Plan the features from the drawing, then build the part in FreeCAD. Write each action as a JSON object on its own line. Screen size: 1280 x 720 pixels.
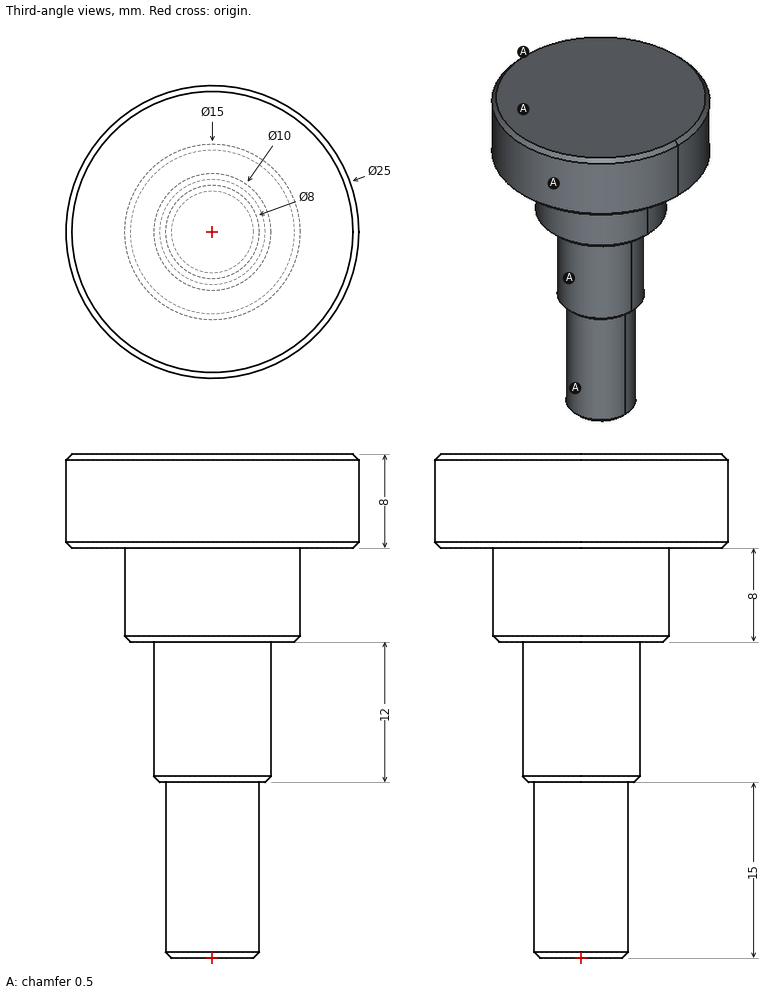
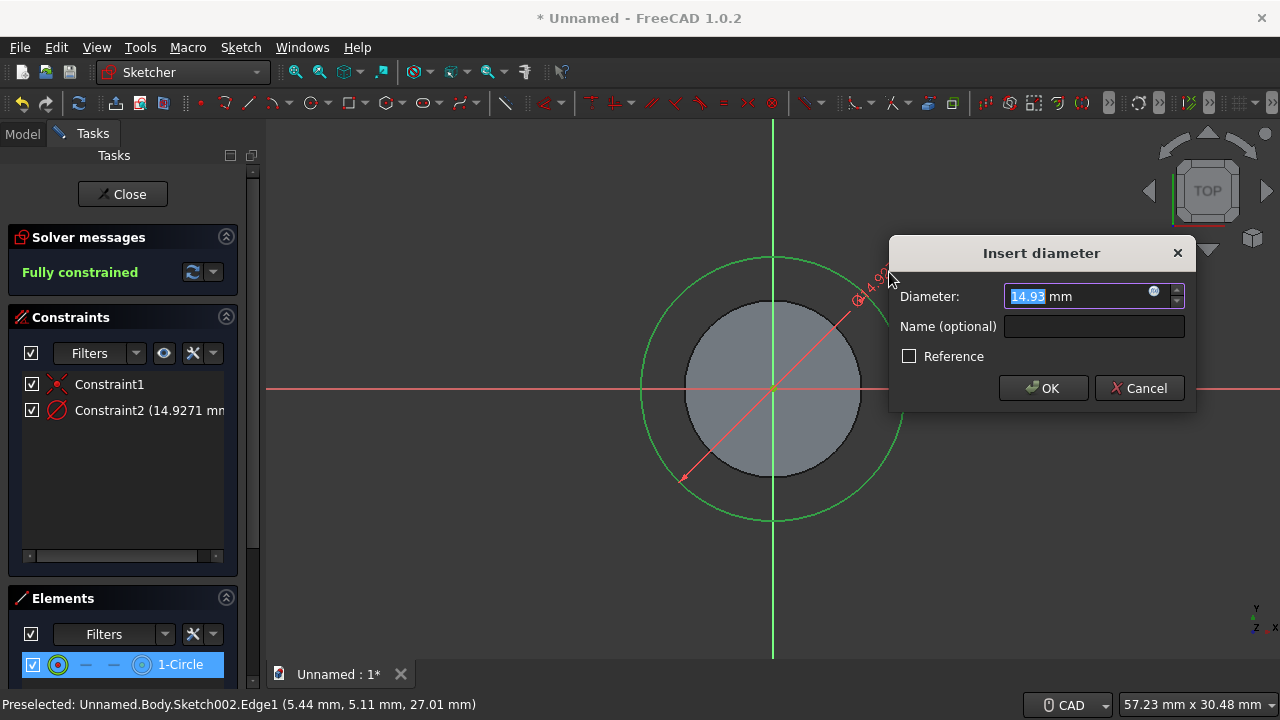
{"action": "type", "text": "15"}
{"action": "key", "text": "Return"}
{"action": "key", "text": "Escape"}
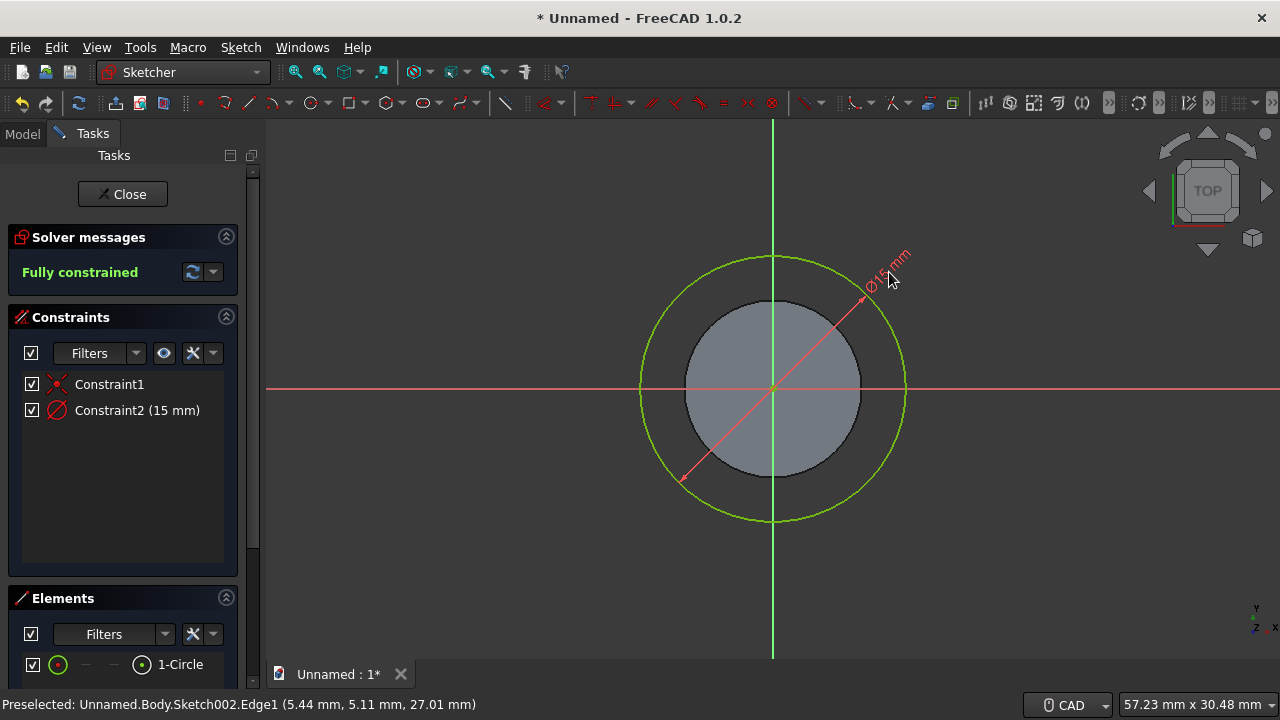
{"action": "left_click", "coordinate": [123, 194]}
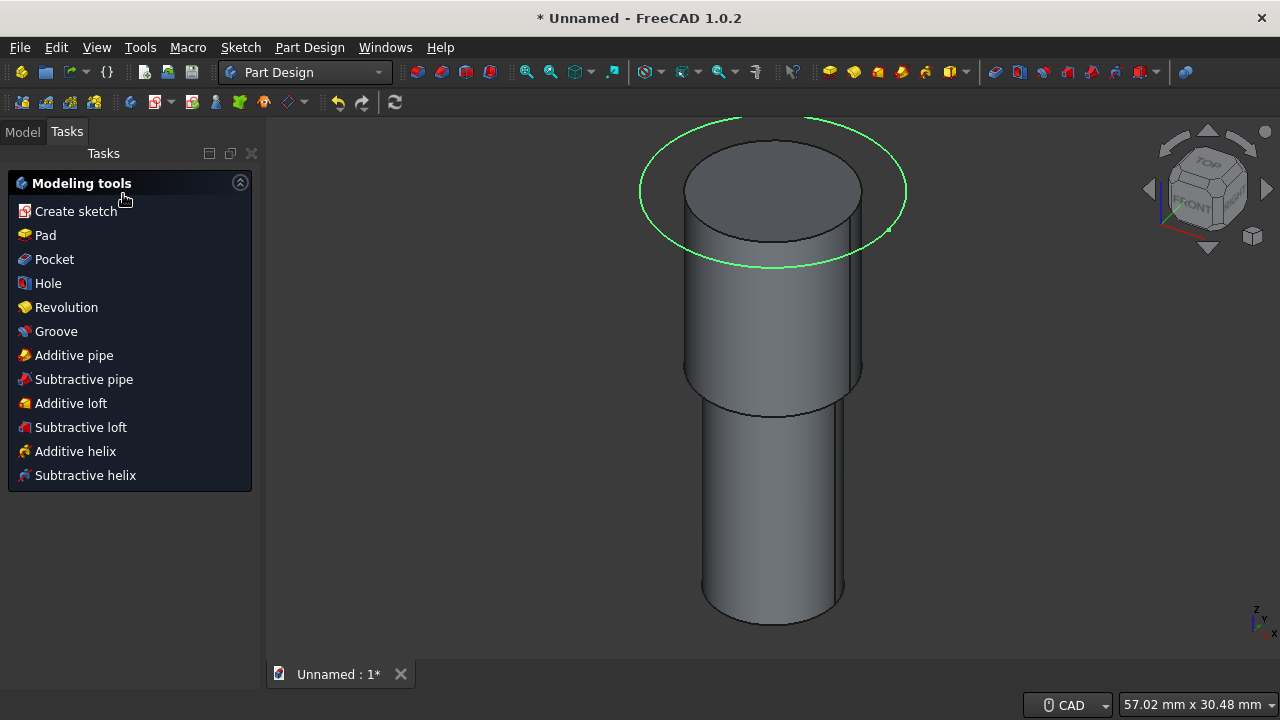
{"action": "left_click", "coordinate": [830, 72]}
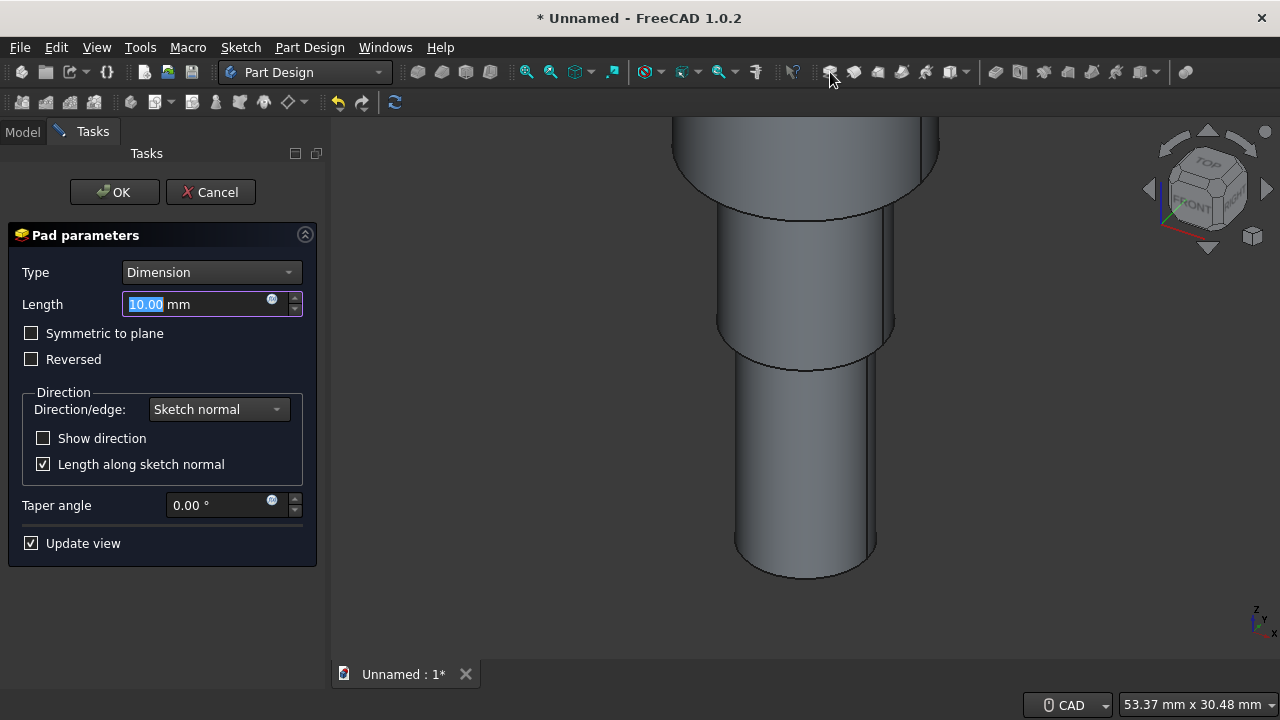
{"action": "type", "text": "8"}
{"action": "key", "text": "Tab"}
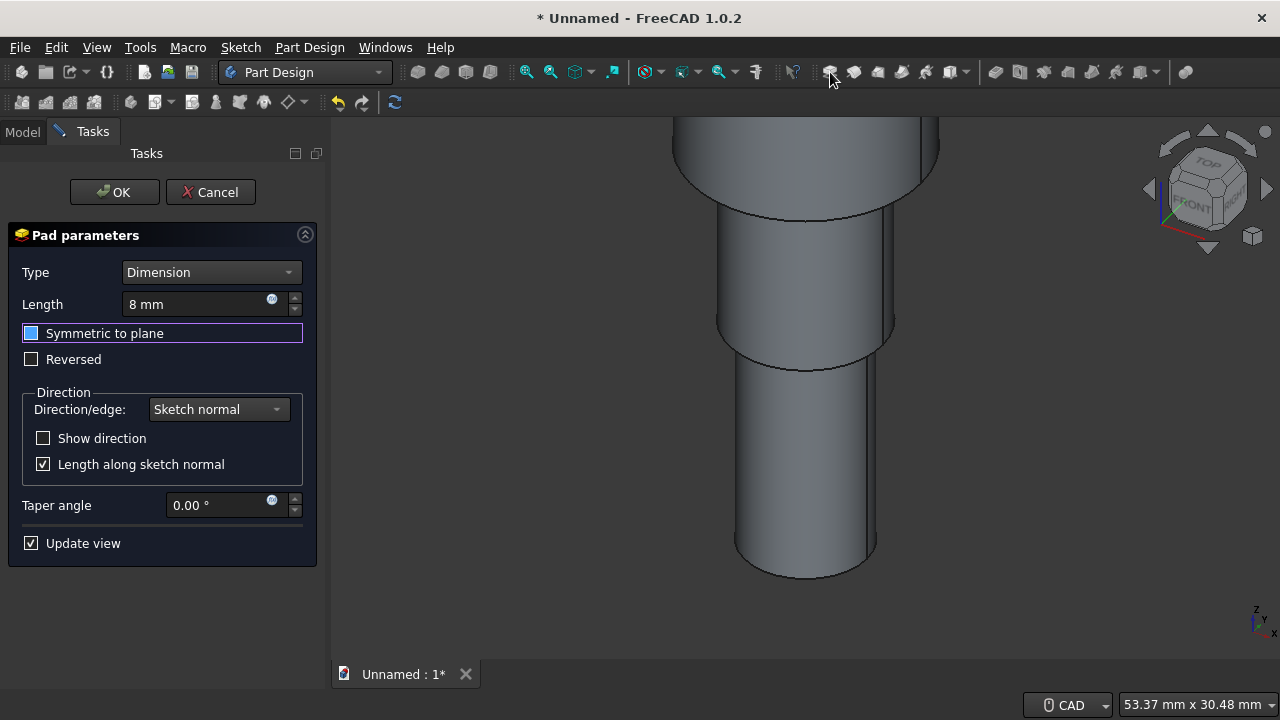
{"action": "left_click", "coordinate": [115, 192]}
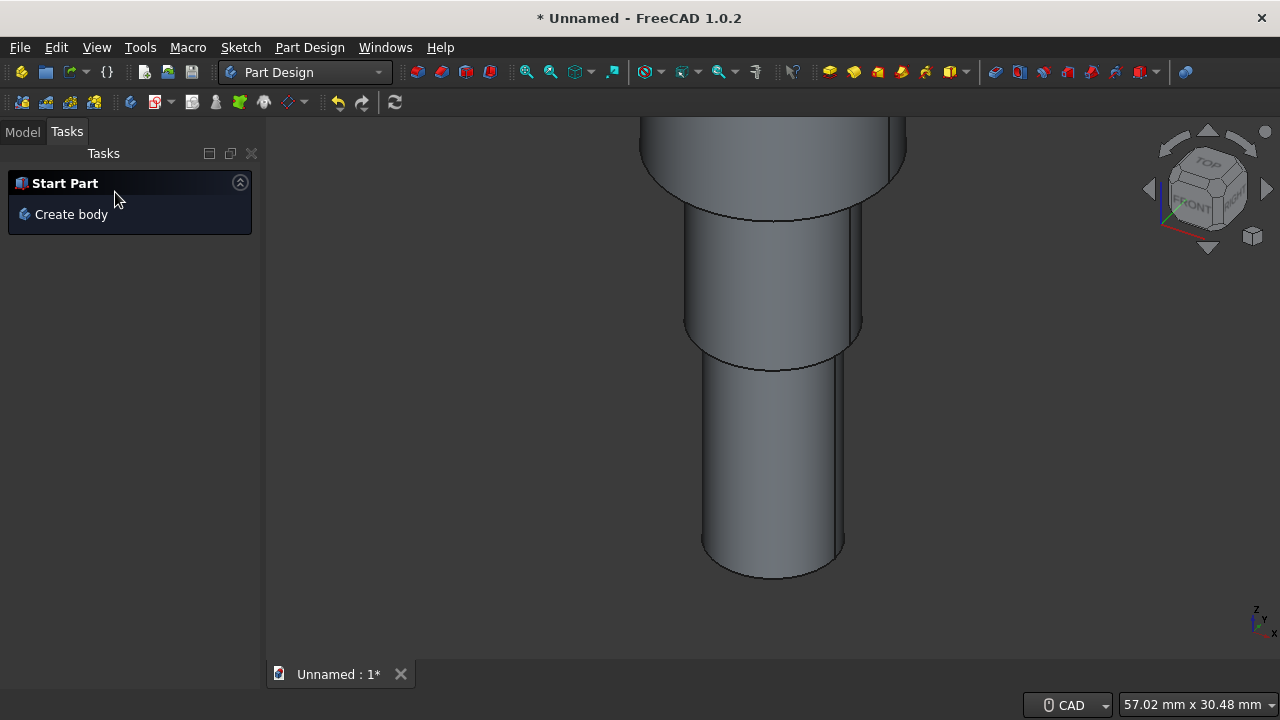
{"action": "left_click", "coordinate": [528, 72]}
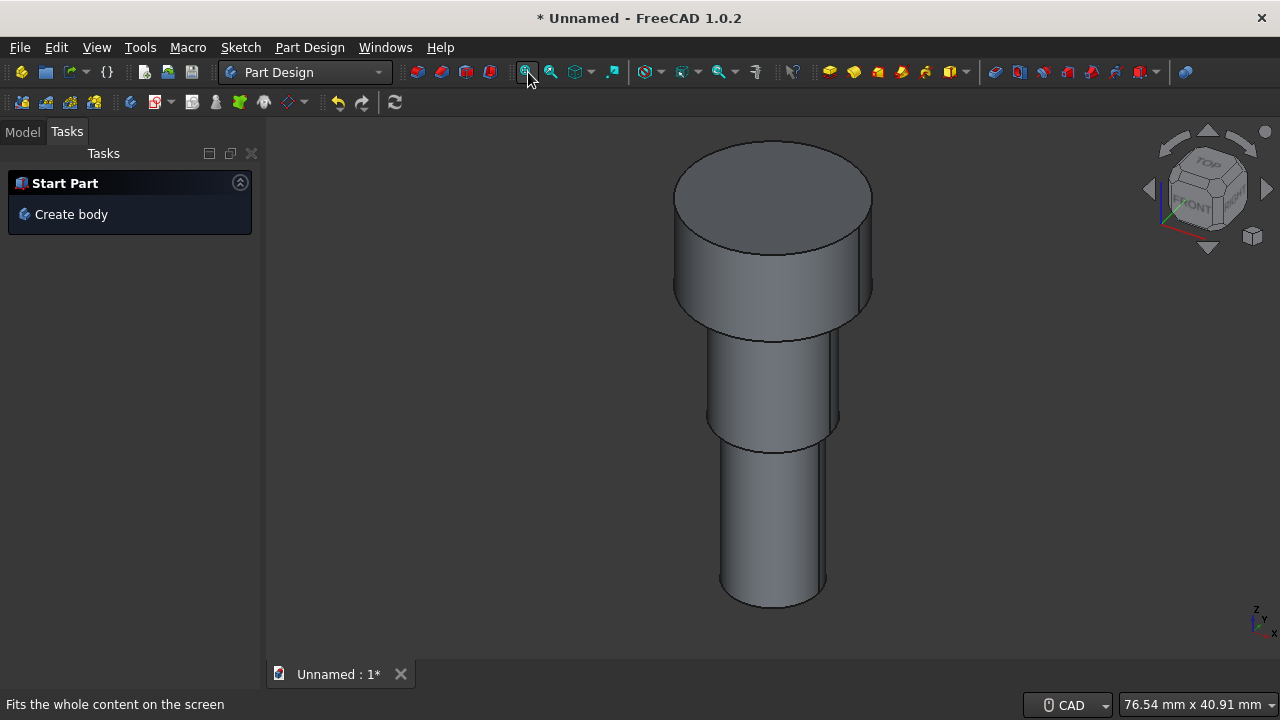
{"action": "left_click", "coordinate": [773, 197]}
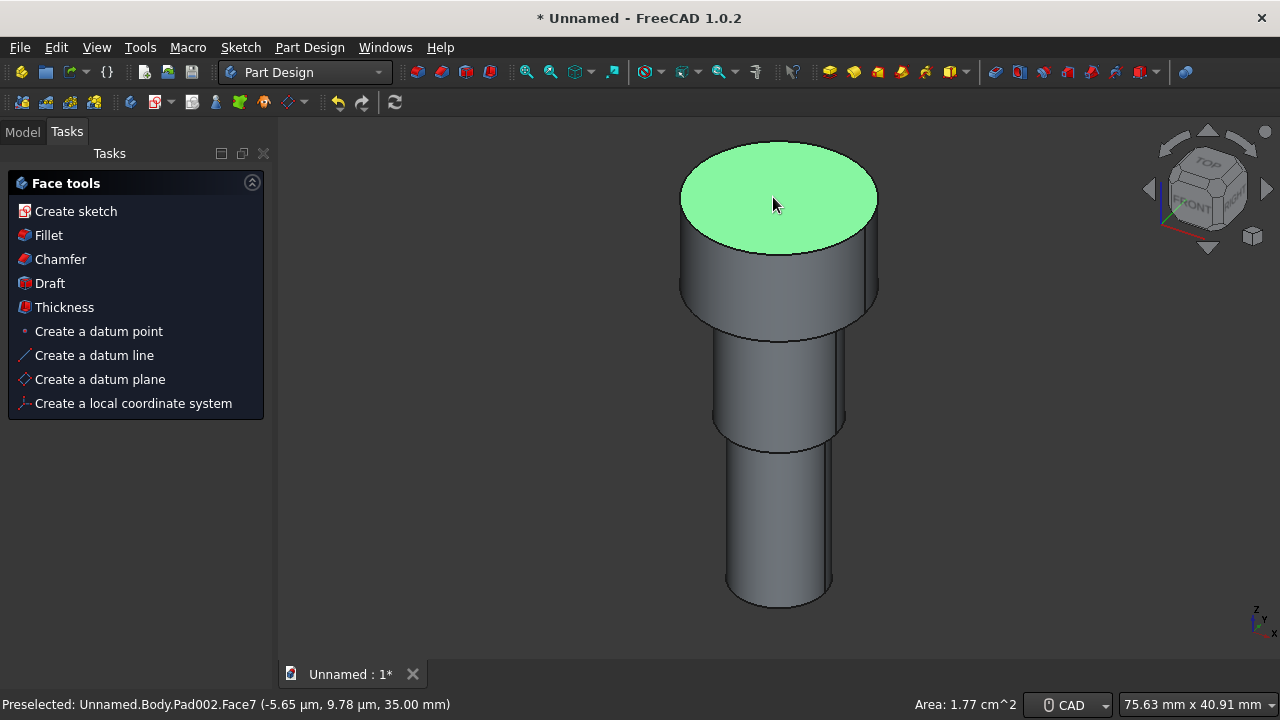
{"action": "left_click", "coordinate": [156, 102]}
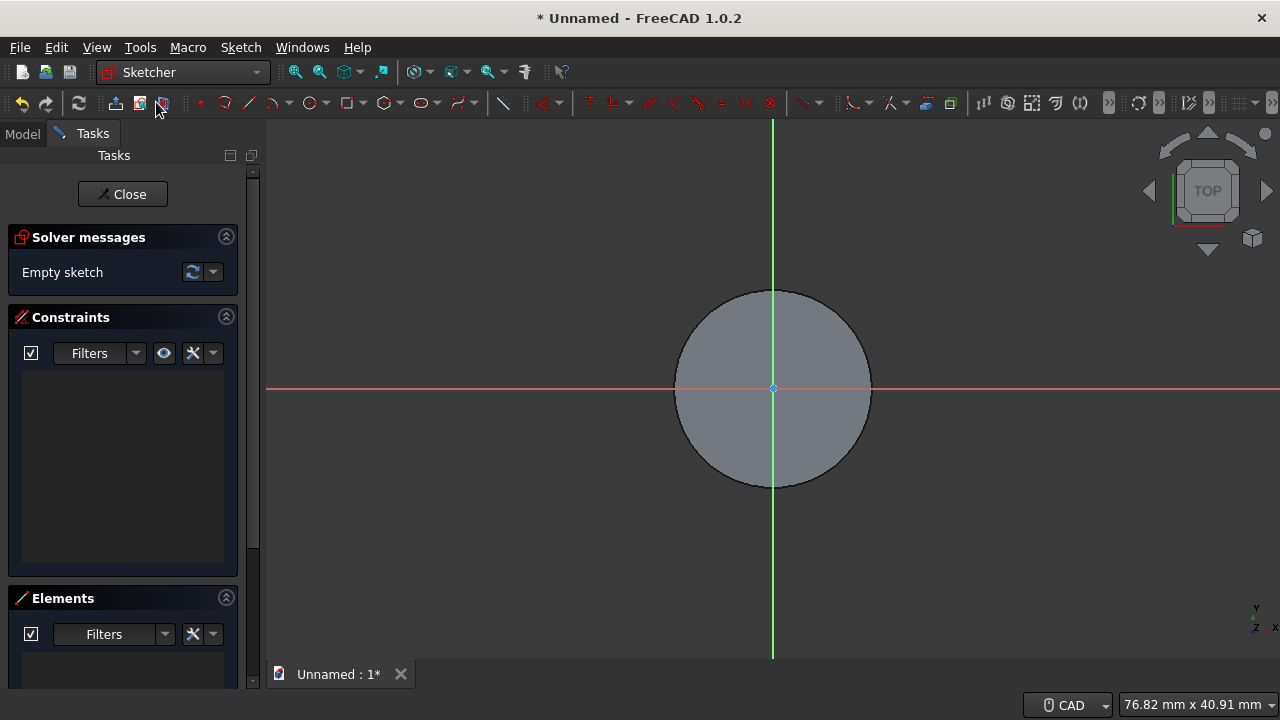
{"action": "left_click", "coordinate": [310, 104]}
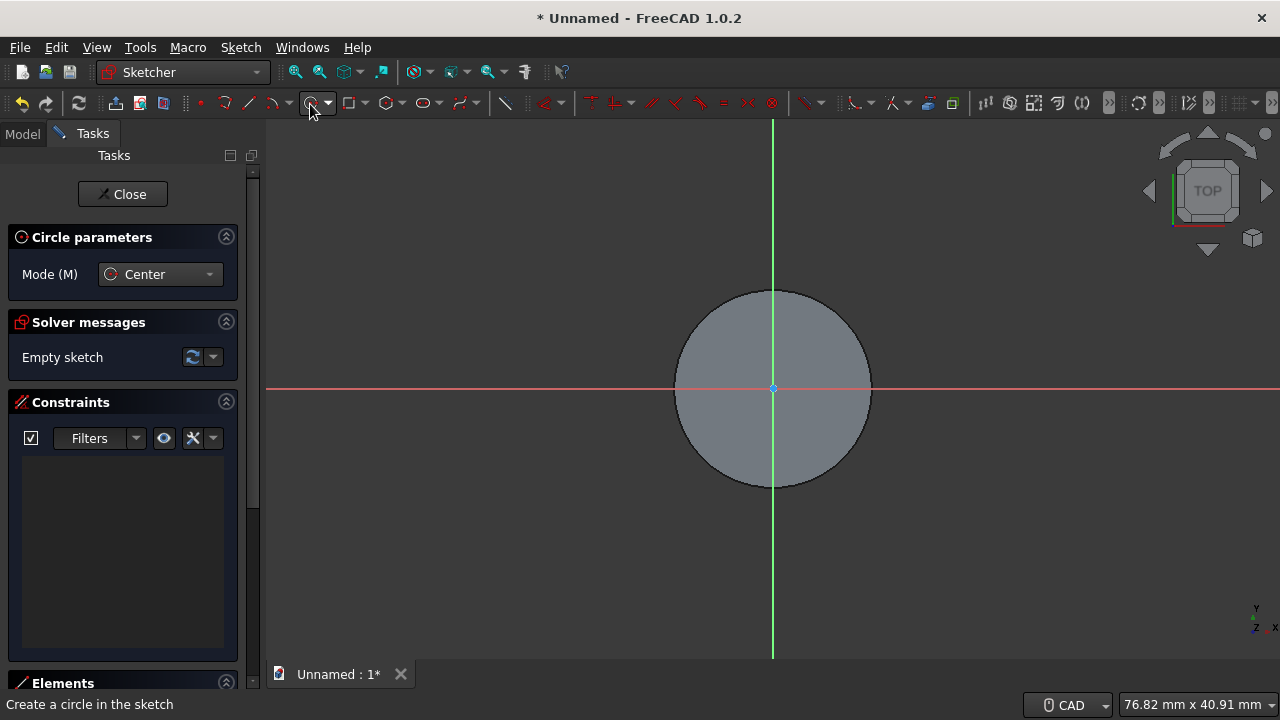
{"action": "left_click", "coordinate": [773, 389]}
{"action": "left_click", "coordinate": [890, 272]}
{"action": "key", "text": "Escape"}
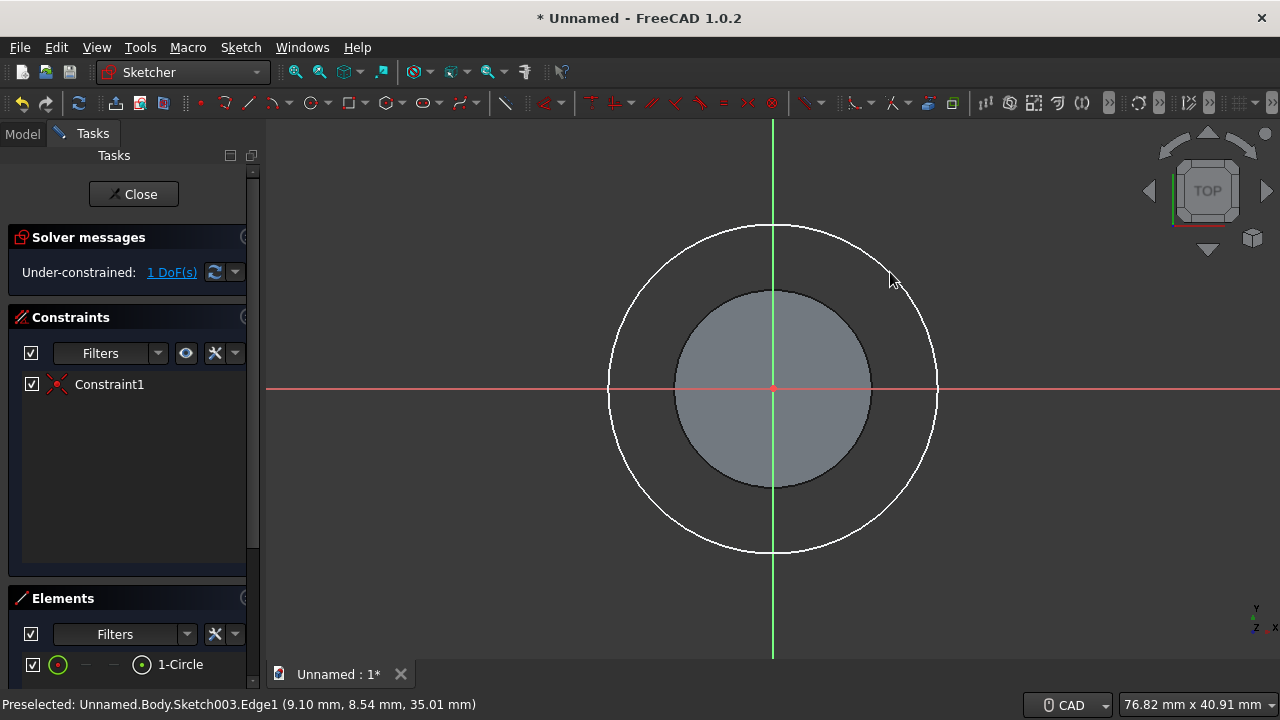
{"action": "left_click", "coordinate": [544, 104]}